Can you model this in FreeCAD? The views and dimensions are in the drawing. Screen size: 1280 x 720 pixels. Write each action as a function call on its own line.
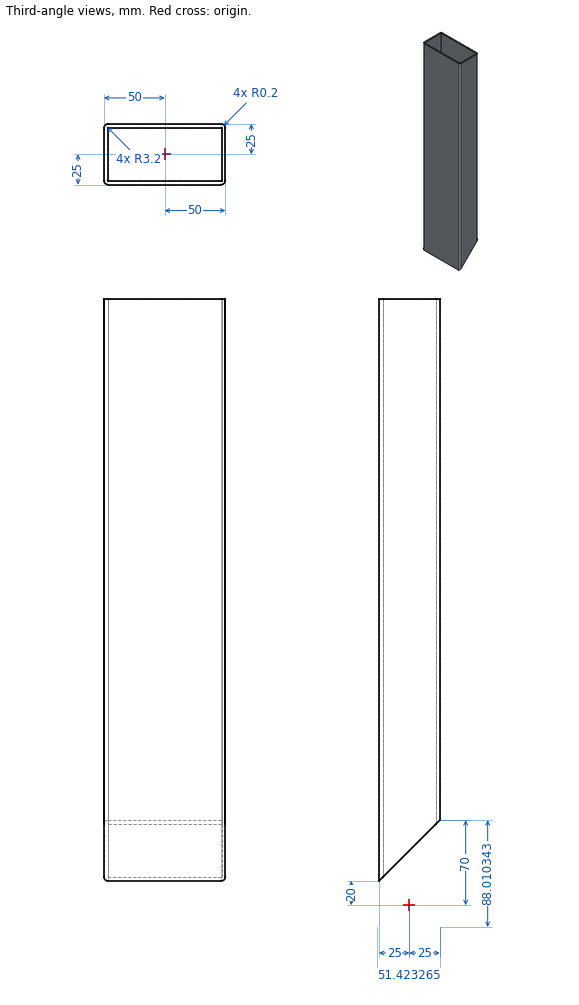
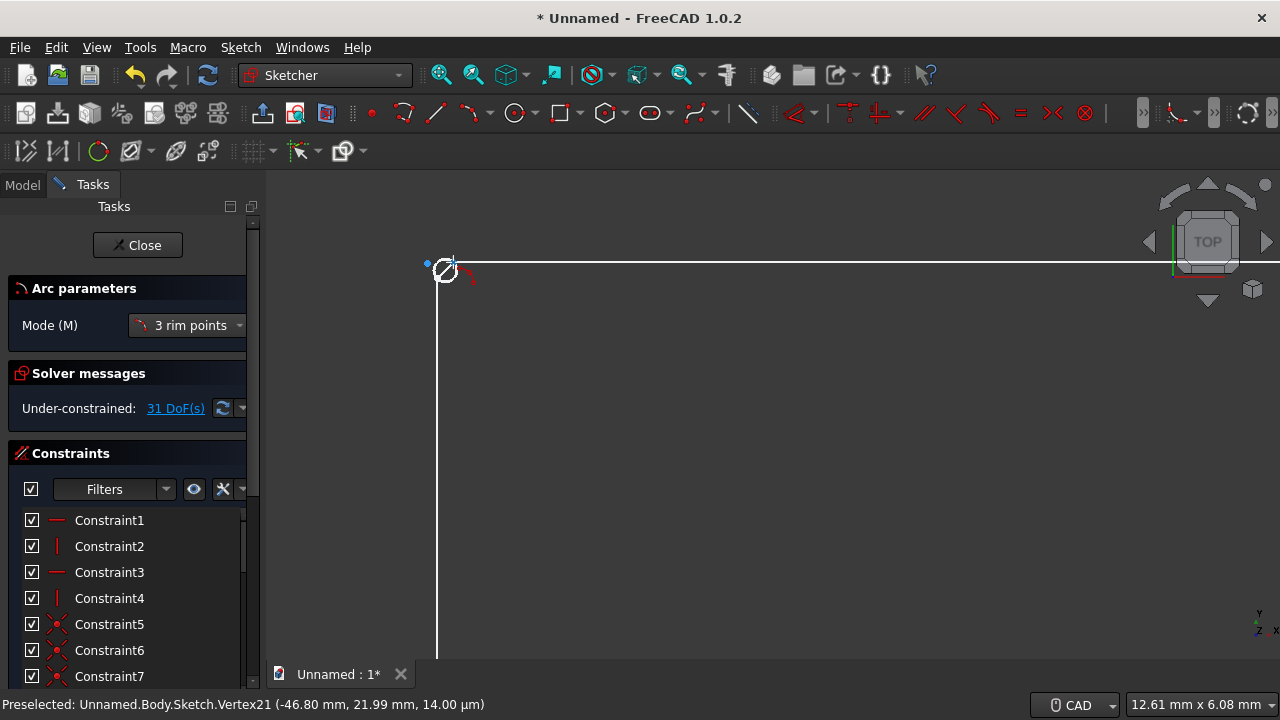
scroll(442, 266, up, 7)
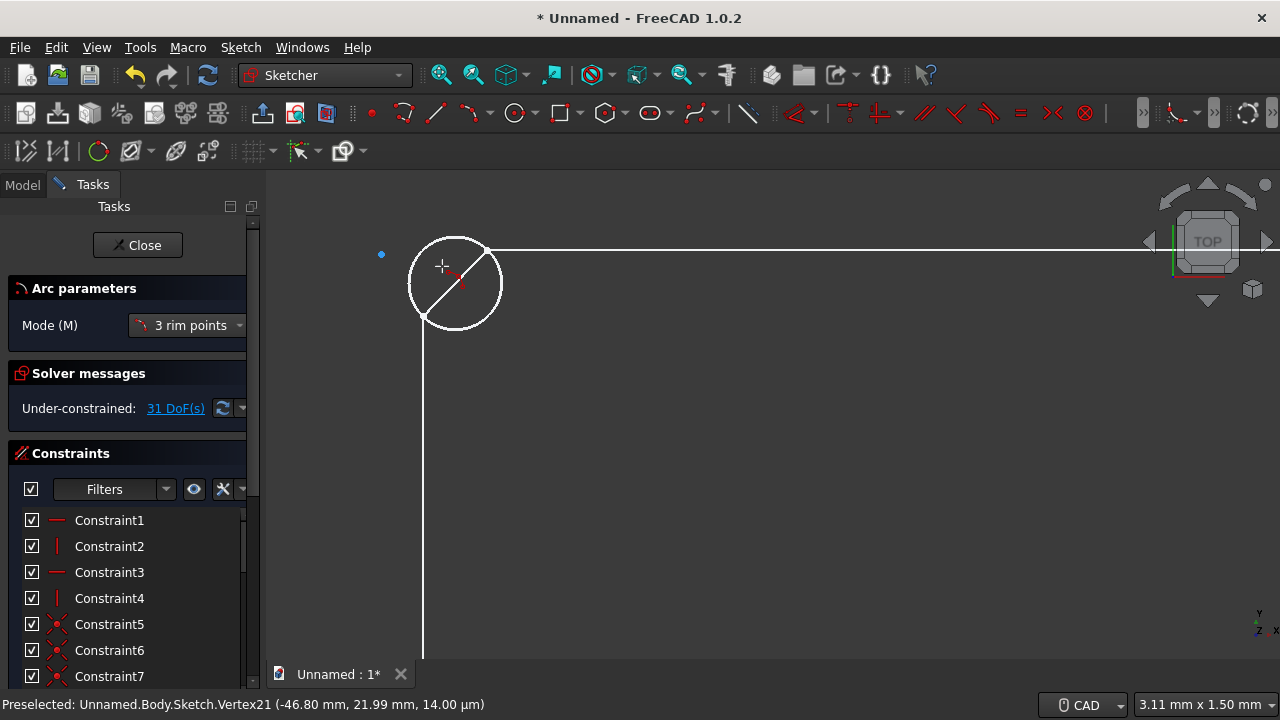
click(441, 265)
key(Escape)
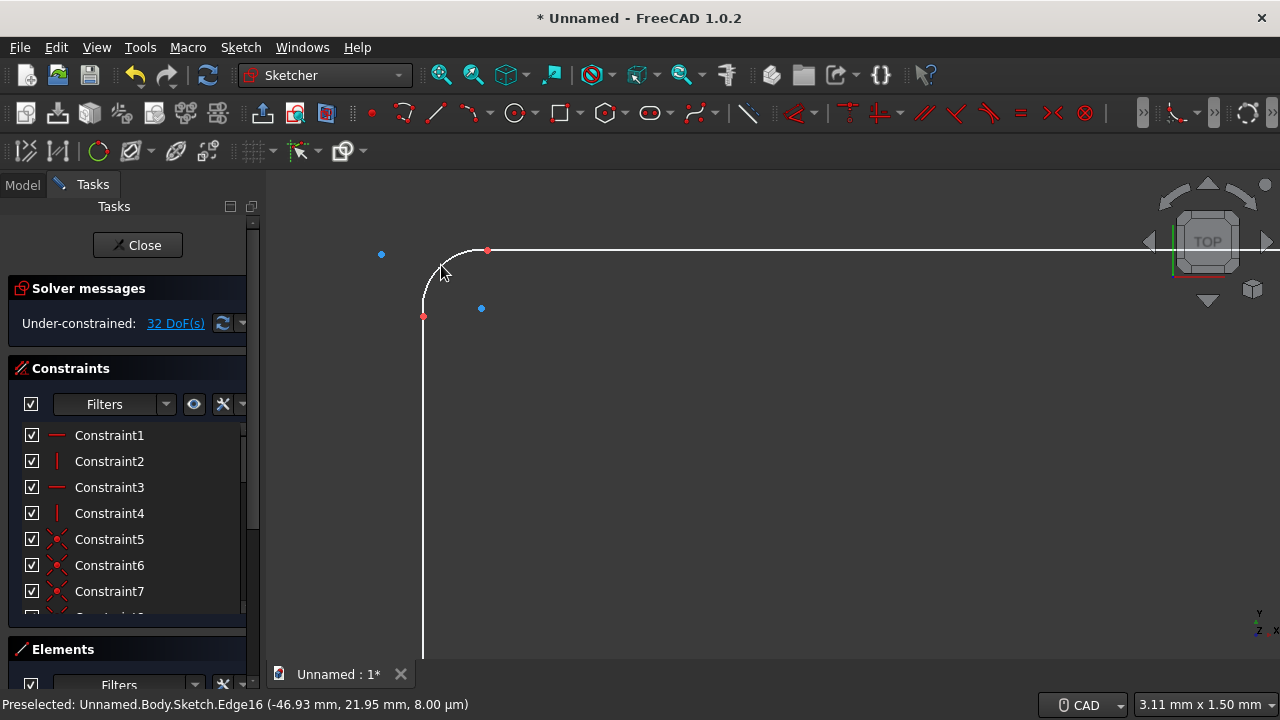
scroll(704, 414, down, 15)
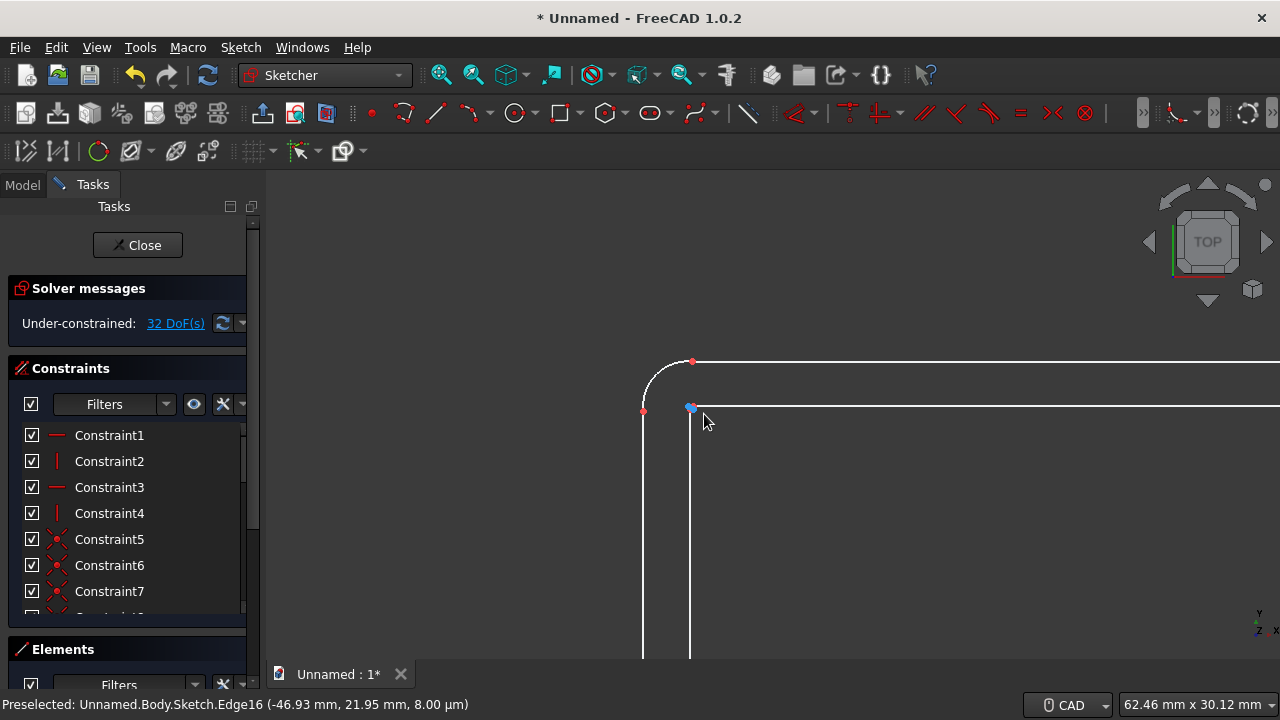
scroll(294, 212, down, 5)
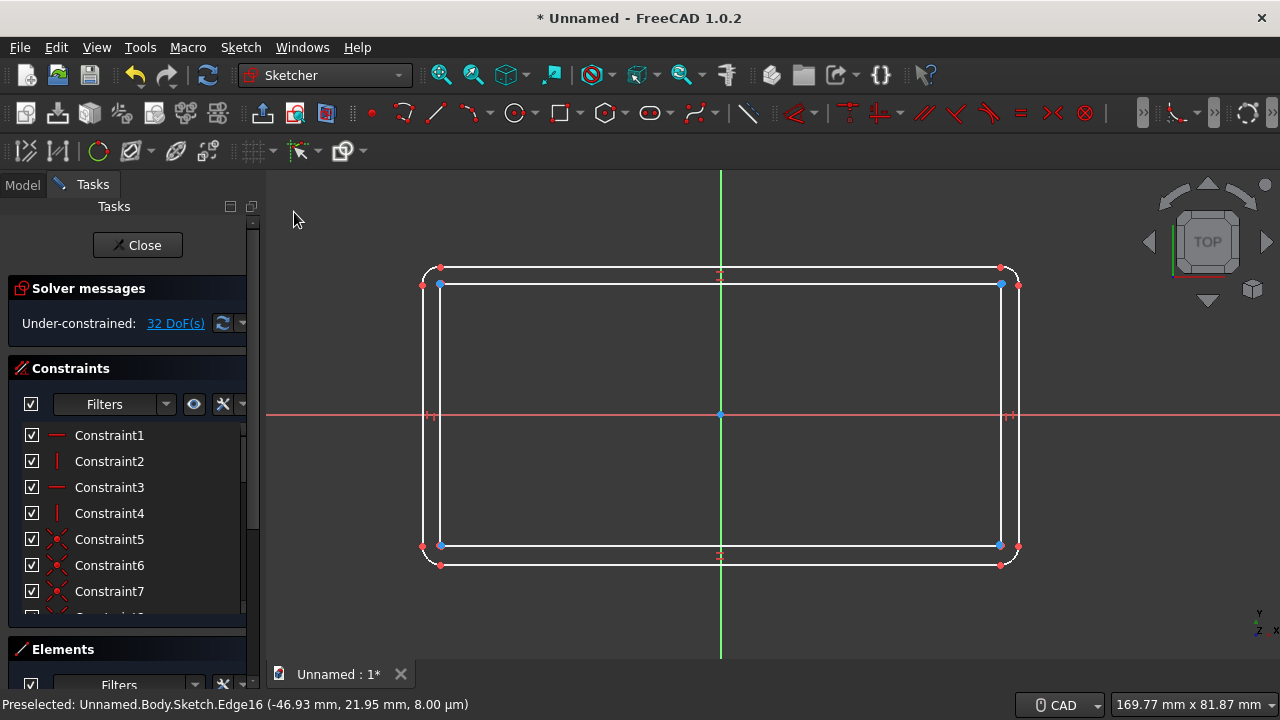
click(832, 267)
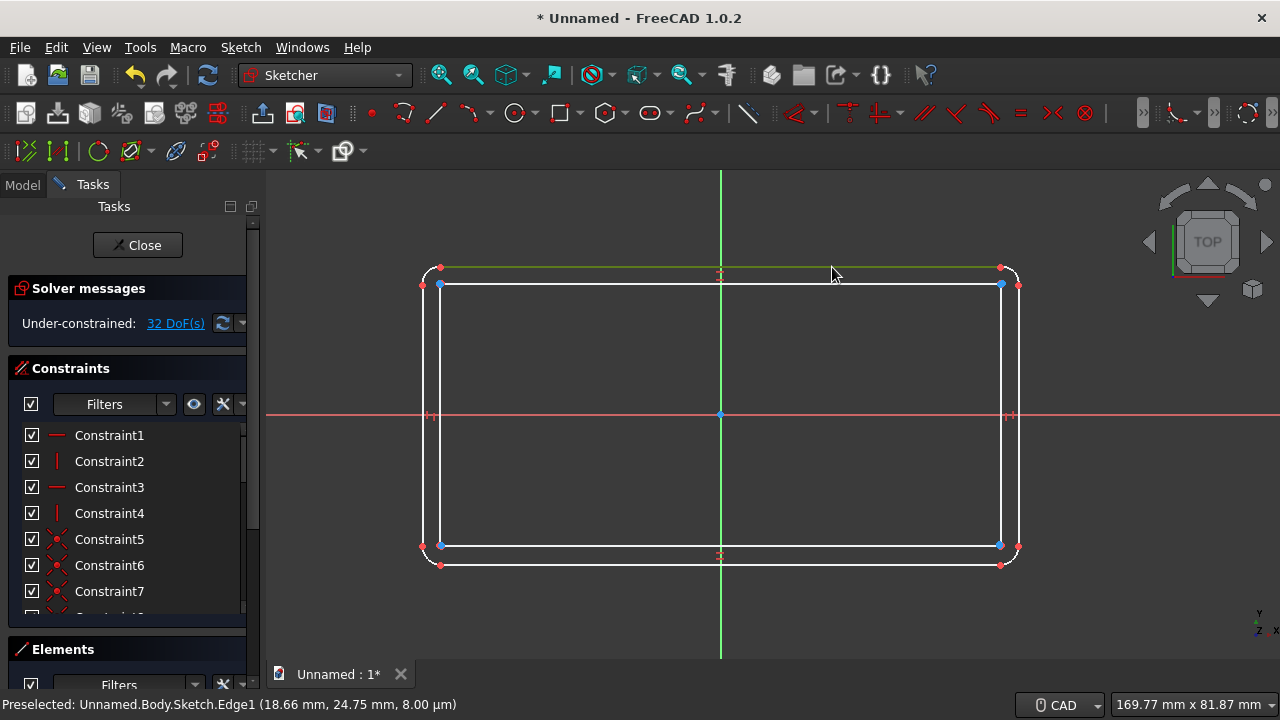
click(427, 272)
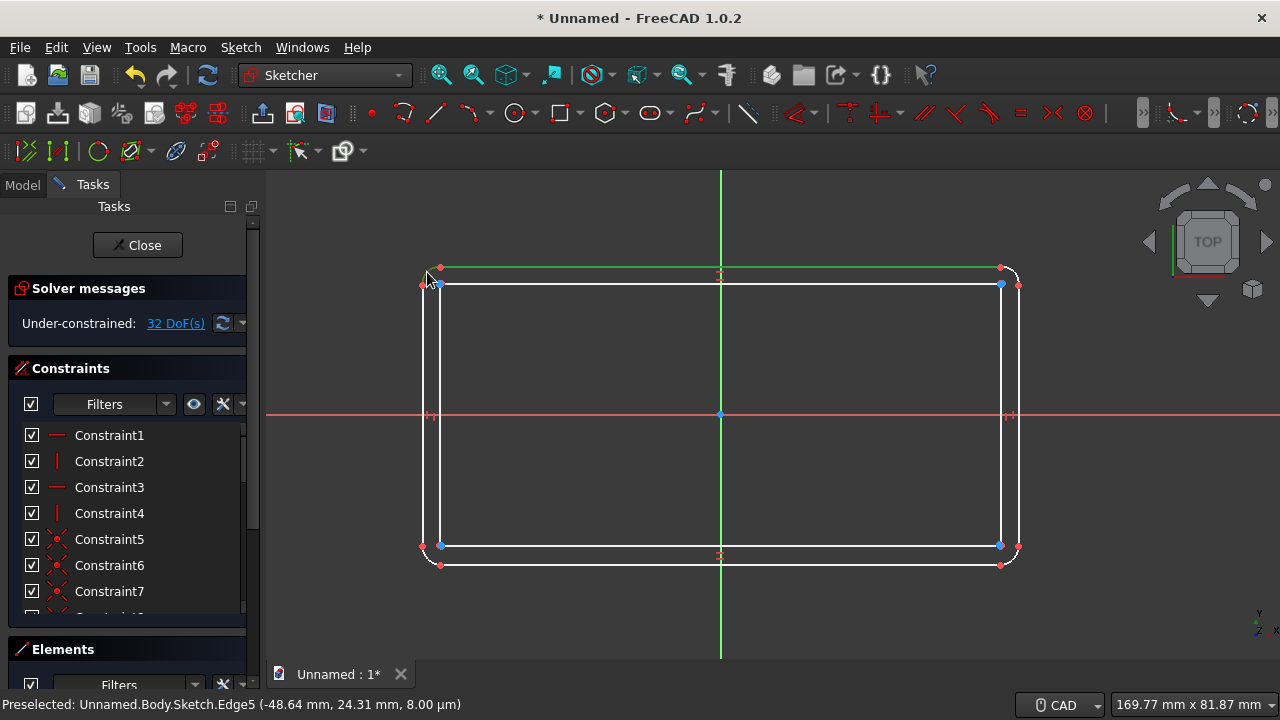
click(990, 114)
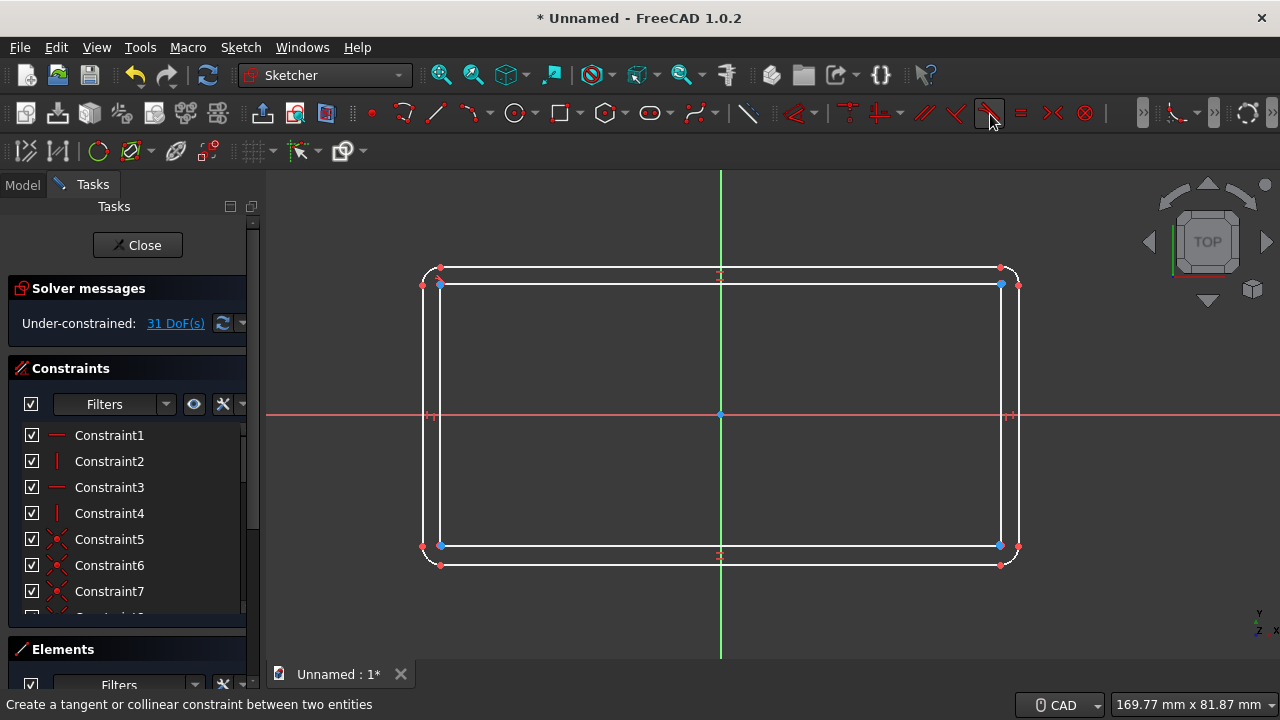
click(832, 267)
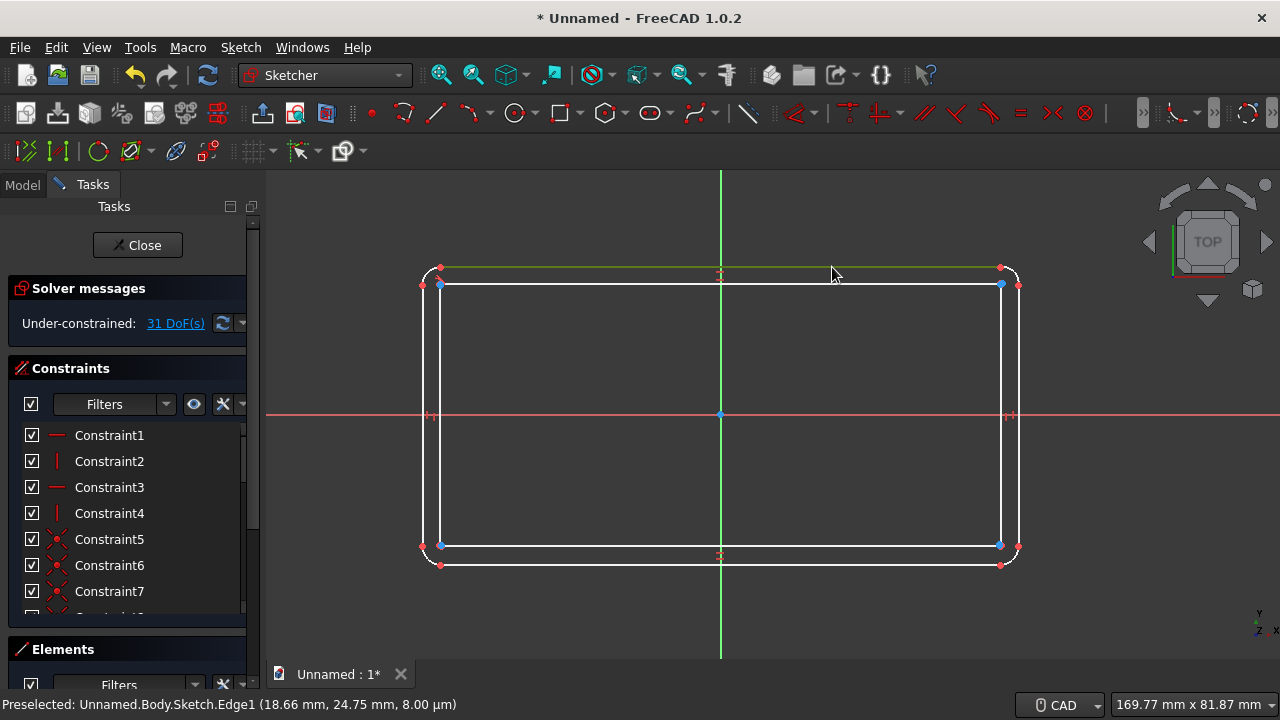
click(1014, 272)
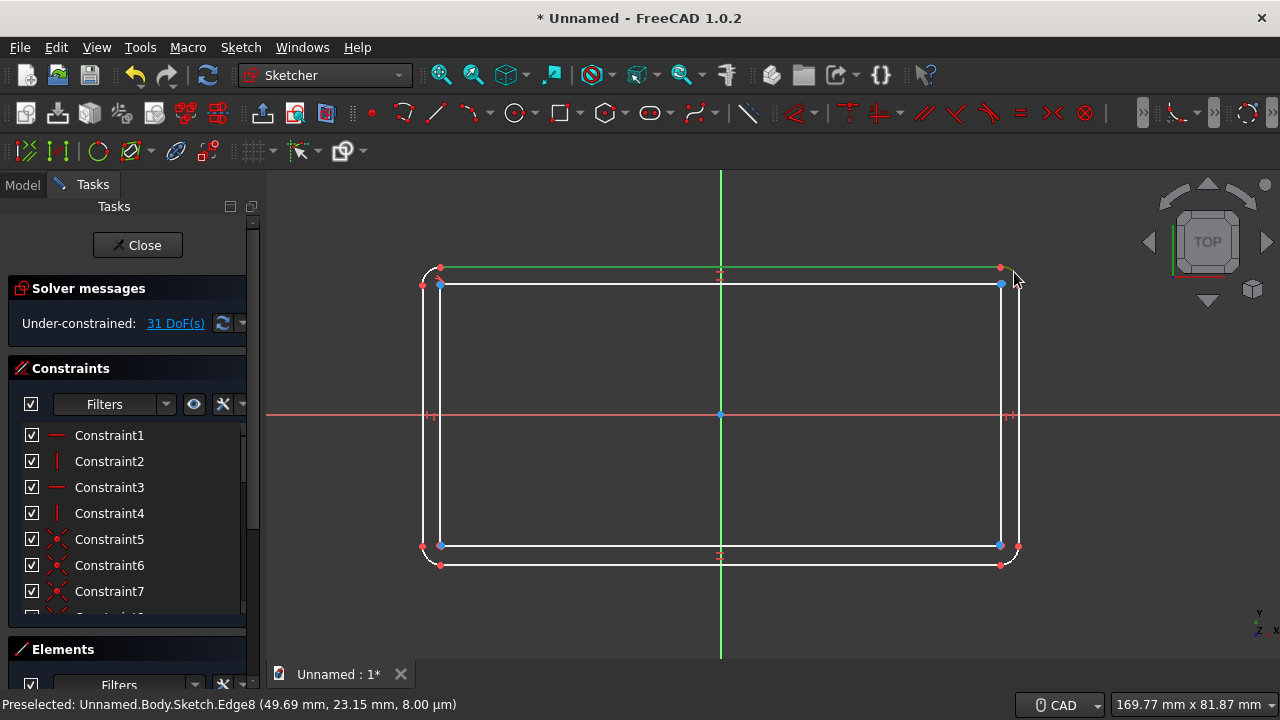
click(990, 114)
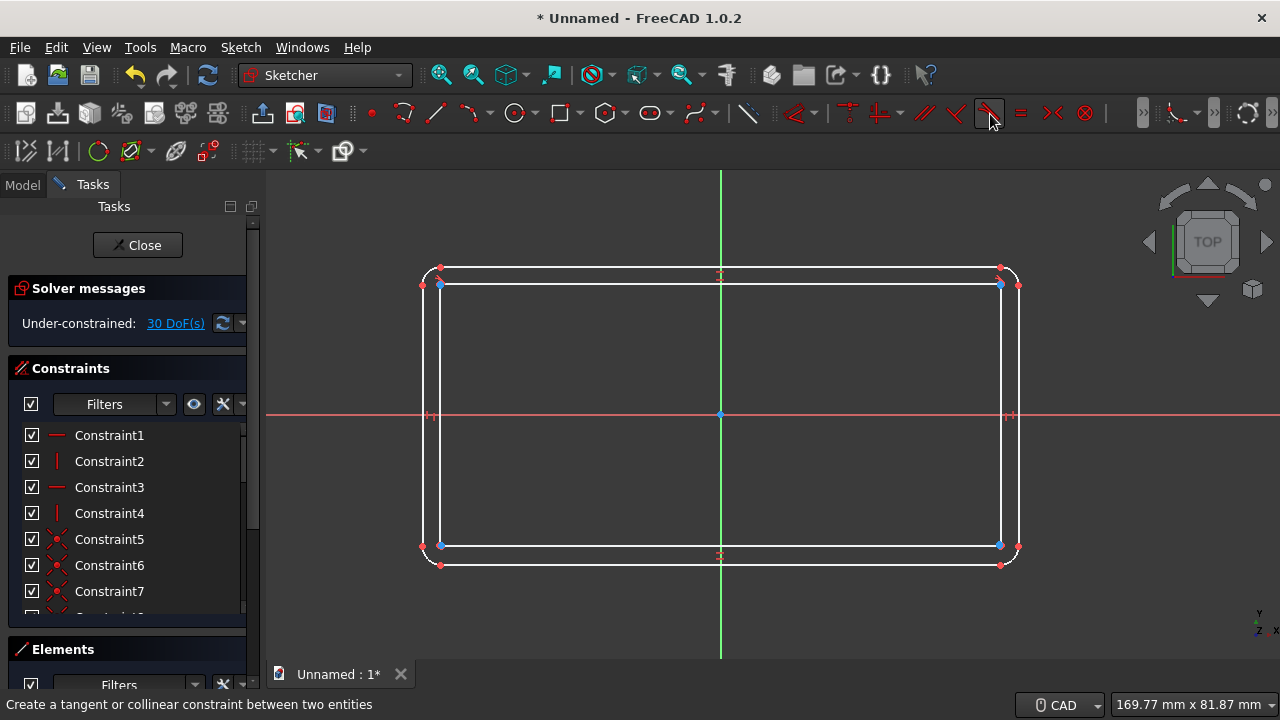
click(423, 364)